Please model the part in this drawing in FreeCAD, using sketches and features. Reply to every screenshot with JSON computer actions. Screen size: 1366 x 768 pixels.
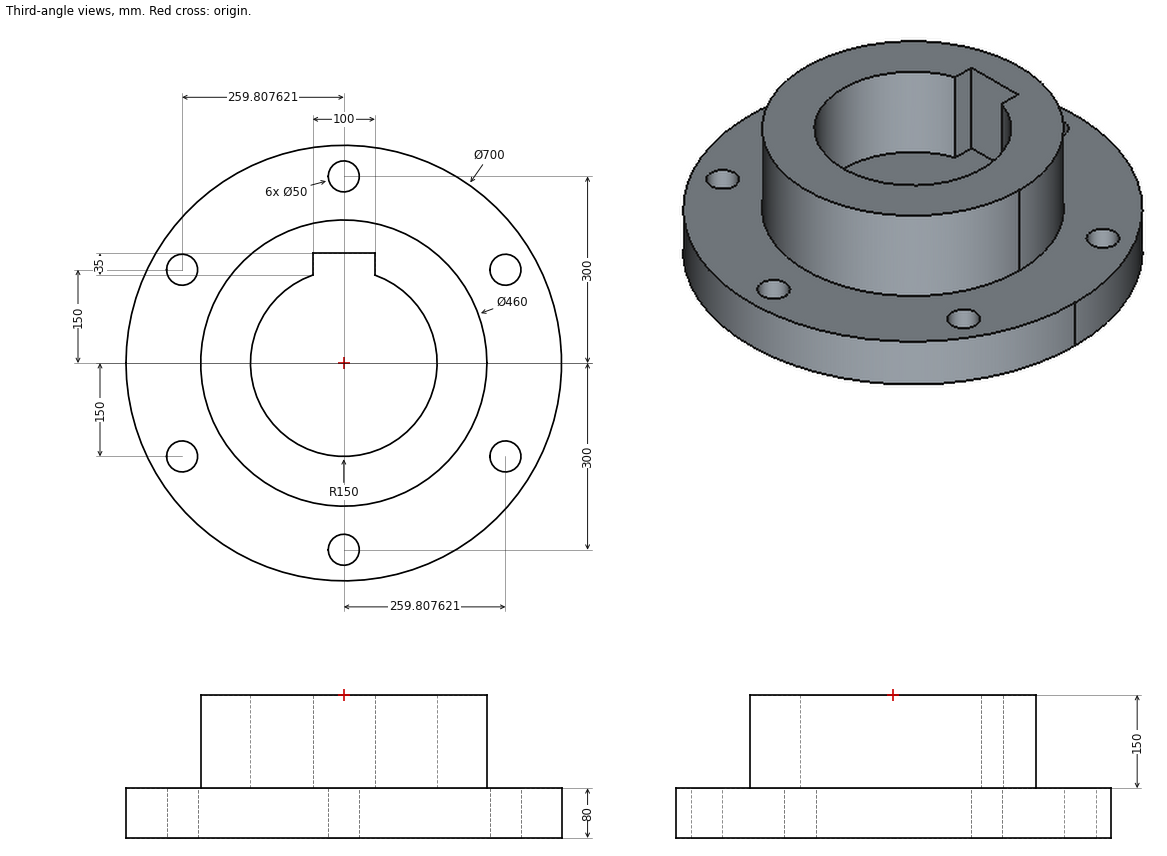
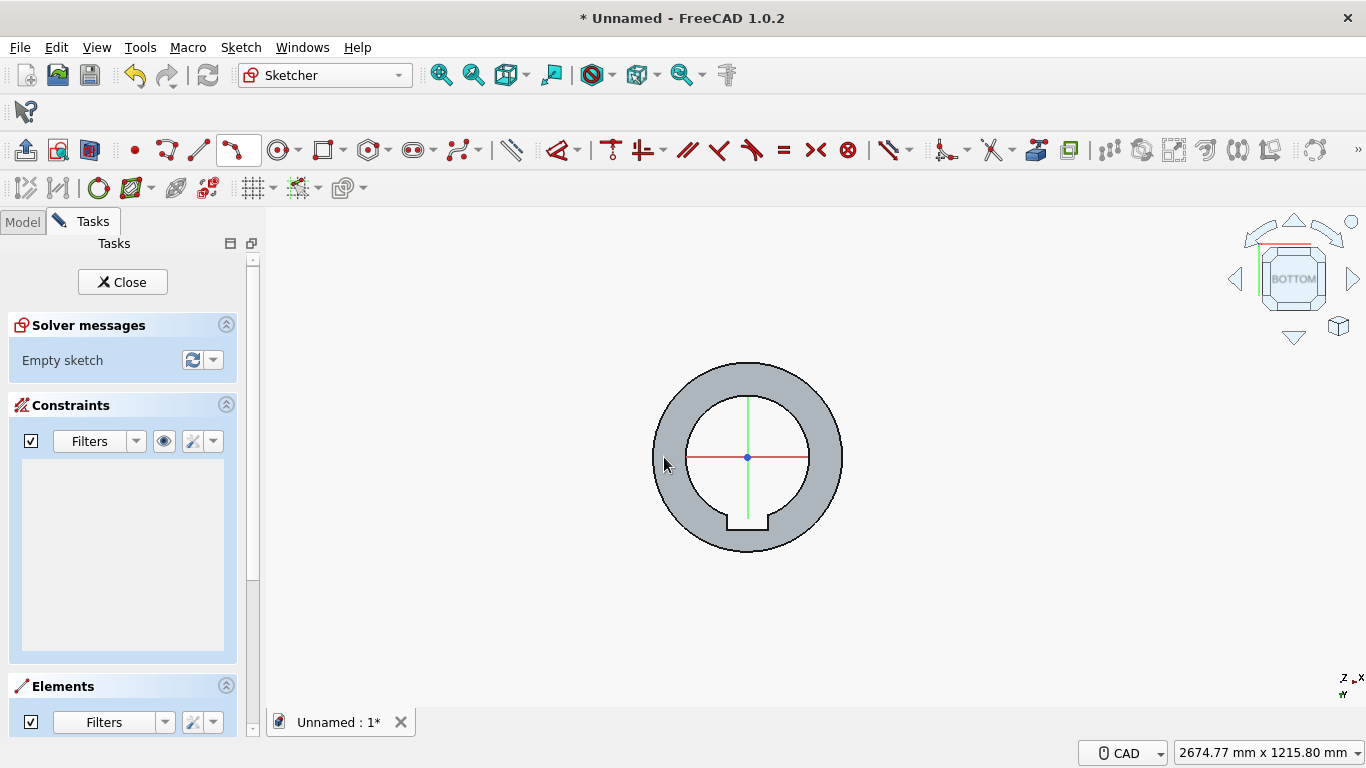
{"action": "left_click", "coordinate": [278, 150]}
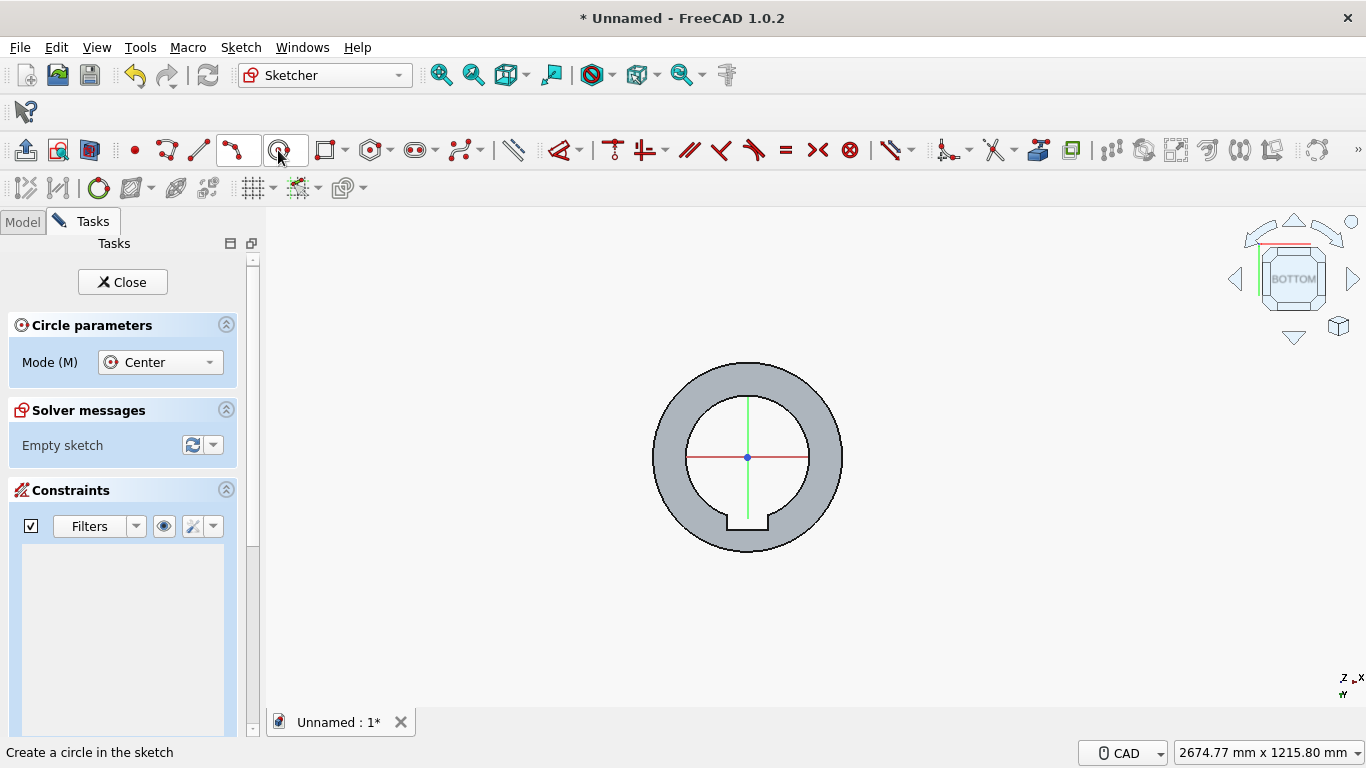
{"action": "left_click", "coordinate": [748, 457]}
{"action": "mouse_move", "coordinate": [849, 355]}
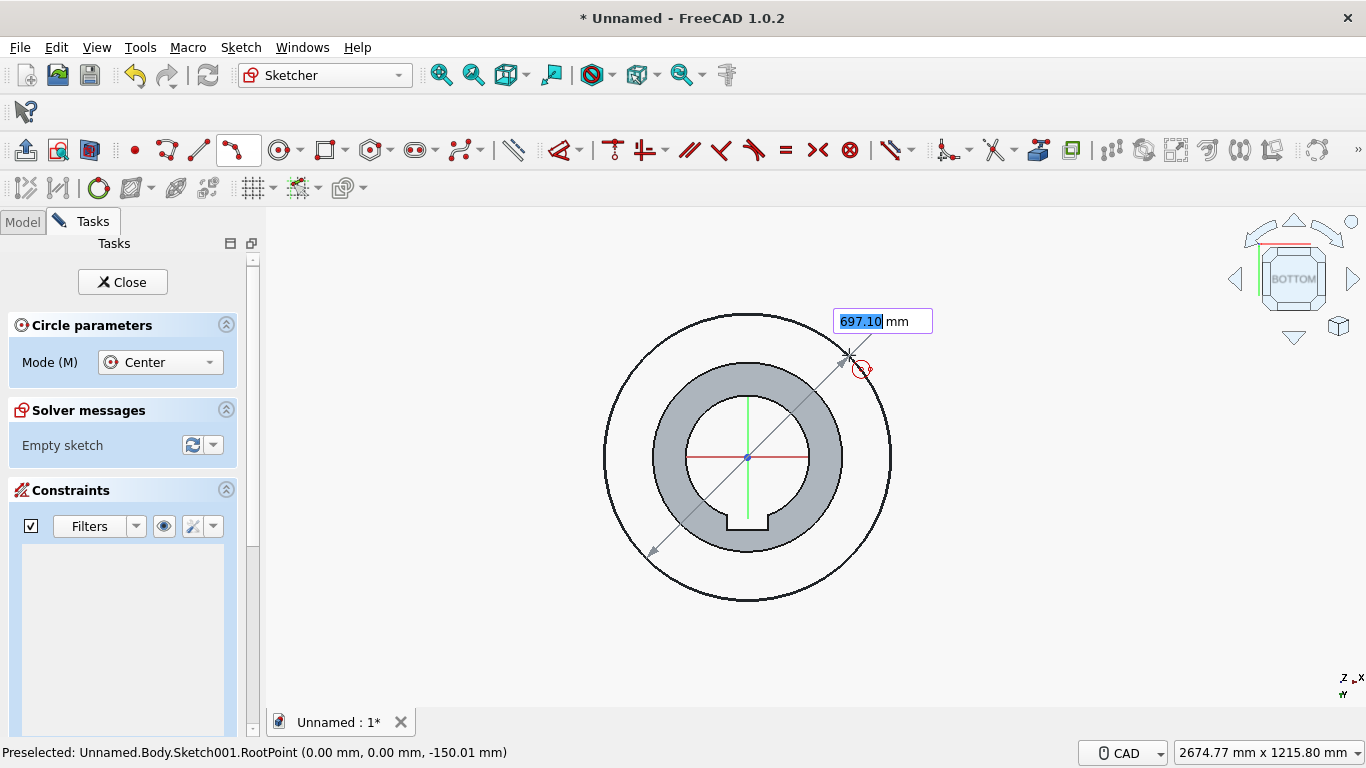
{"action": "type", "text": "700"}
{"action": "key", "text": "Return"}
{"action": "key", "text": "Escape"}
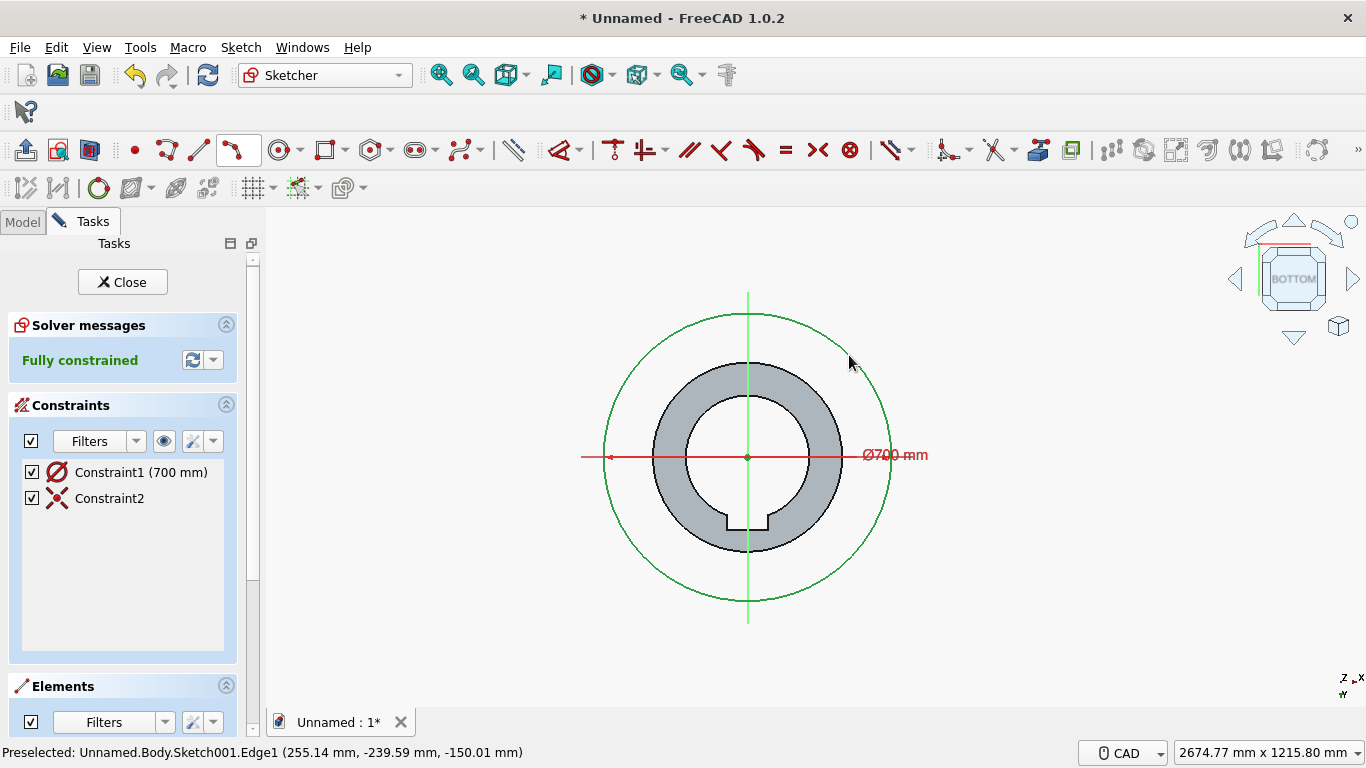
{"action": "left_click", "coordinate": [123, 282]}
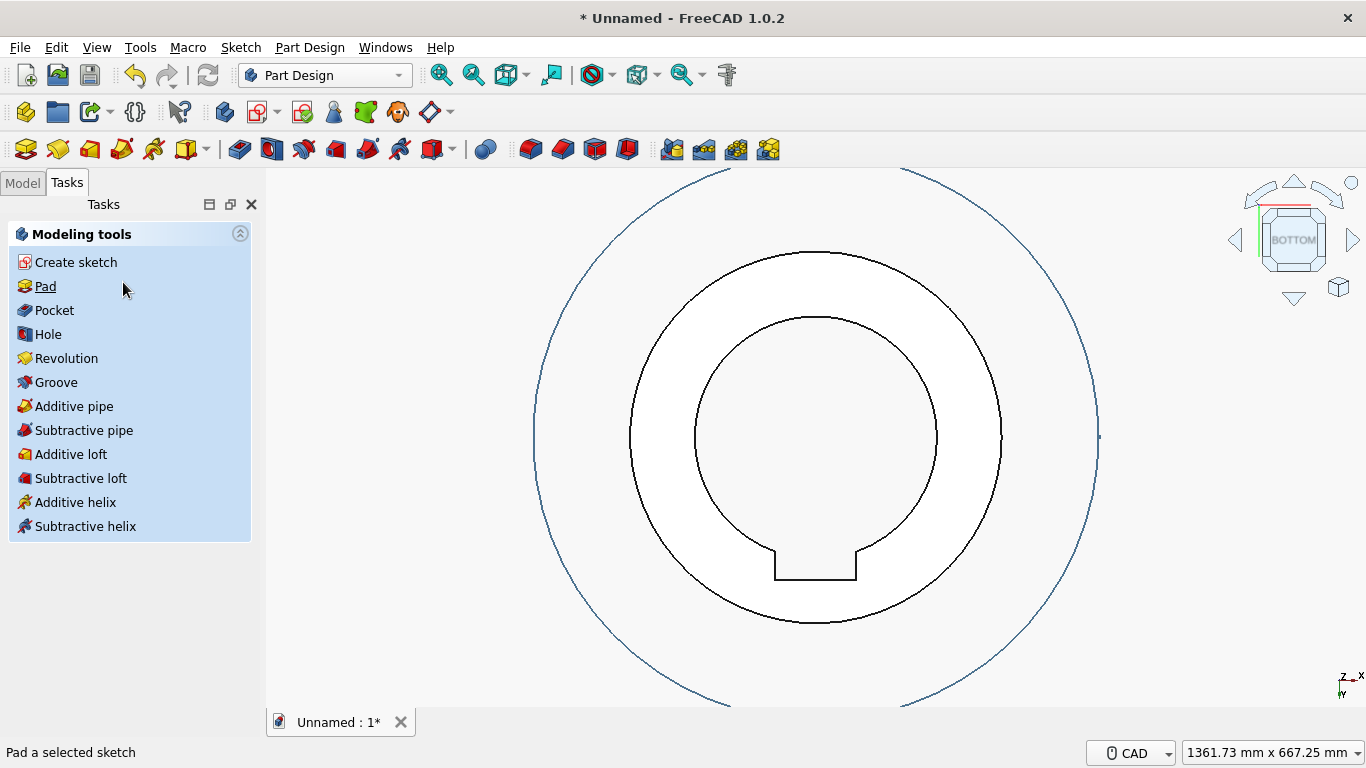
{"action": "left_click", "coordinate": [26, 150]}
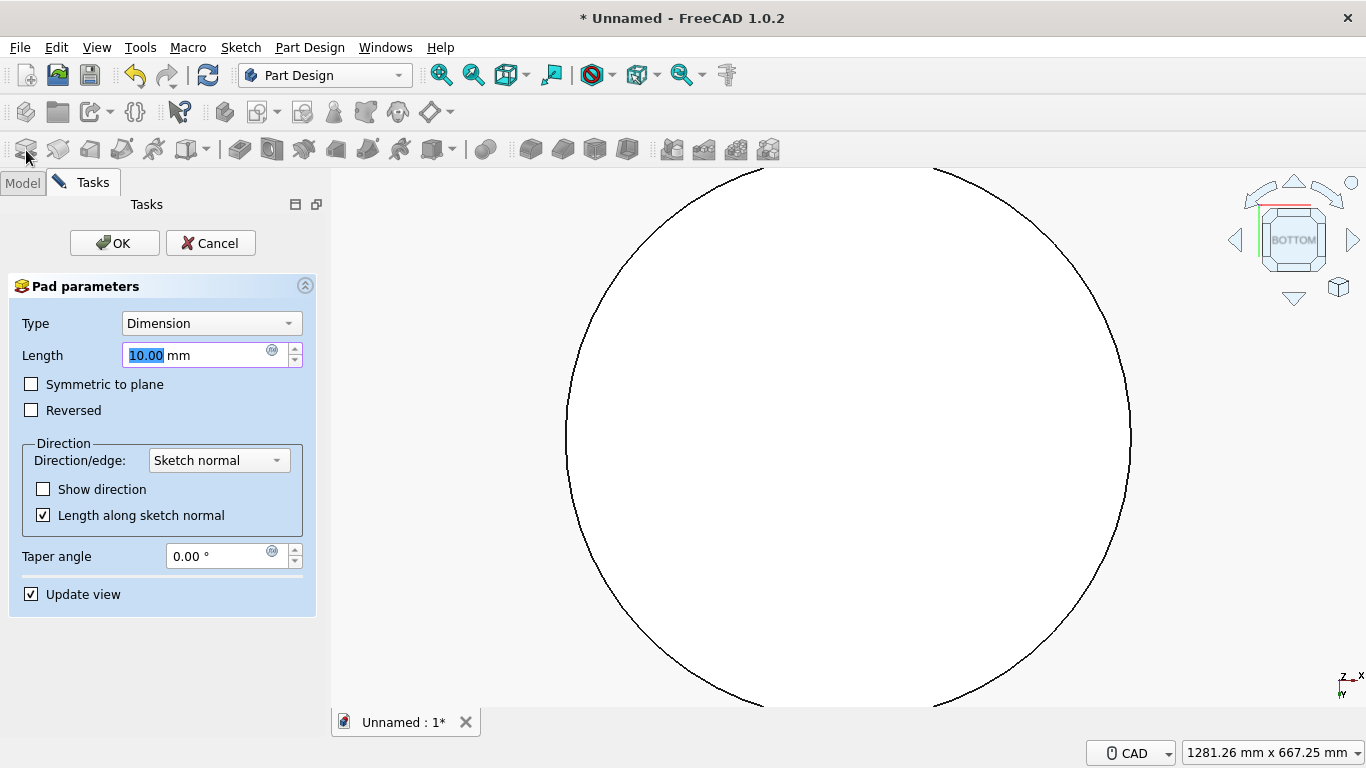
{"action": "type", "text": "80"}
{"action": "key", "text": "Tab"}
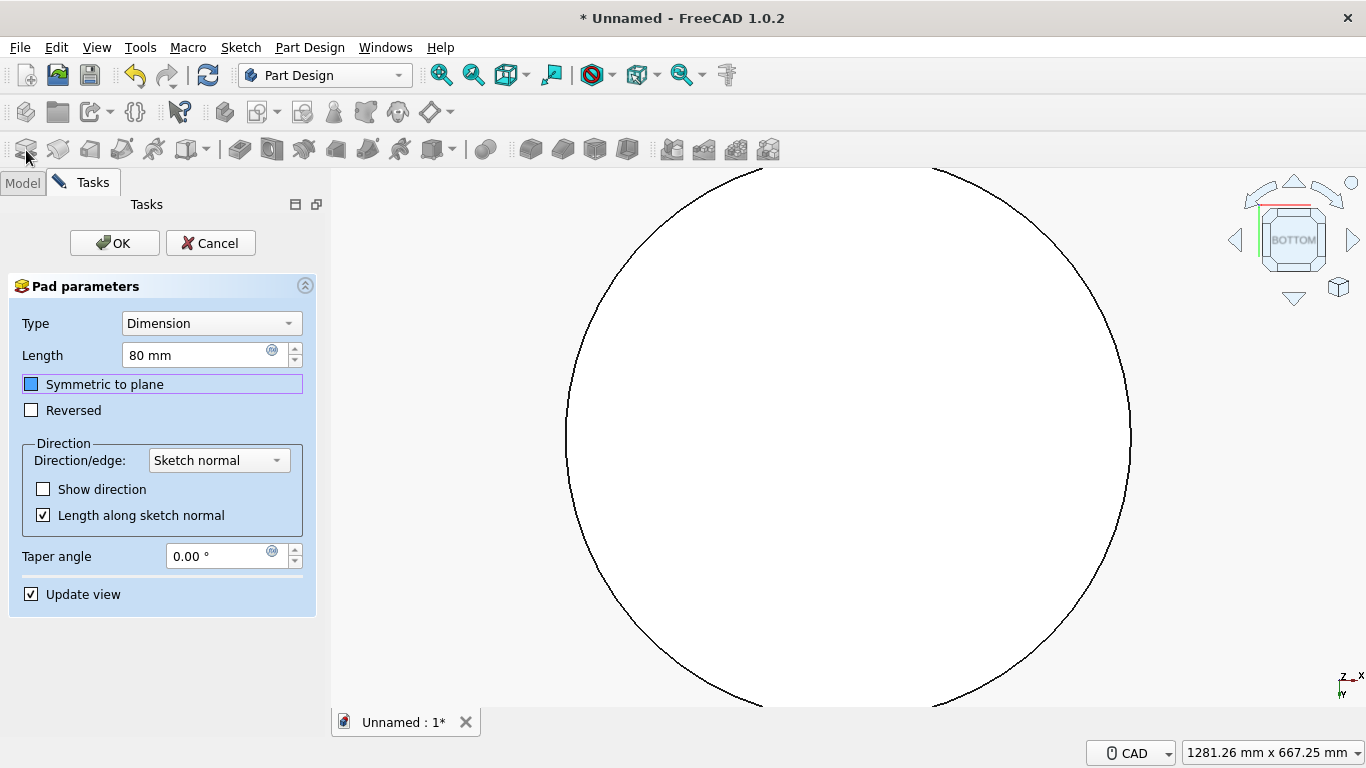
{"action": "left_click", "coordinate": [115, 243]}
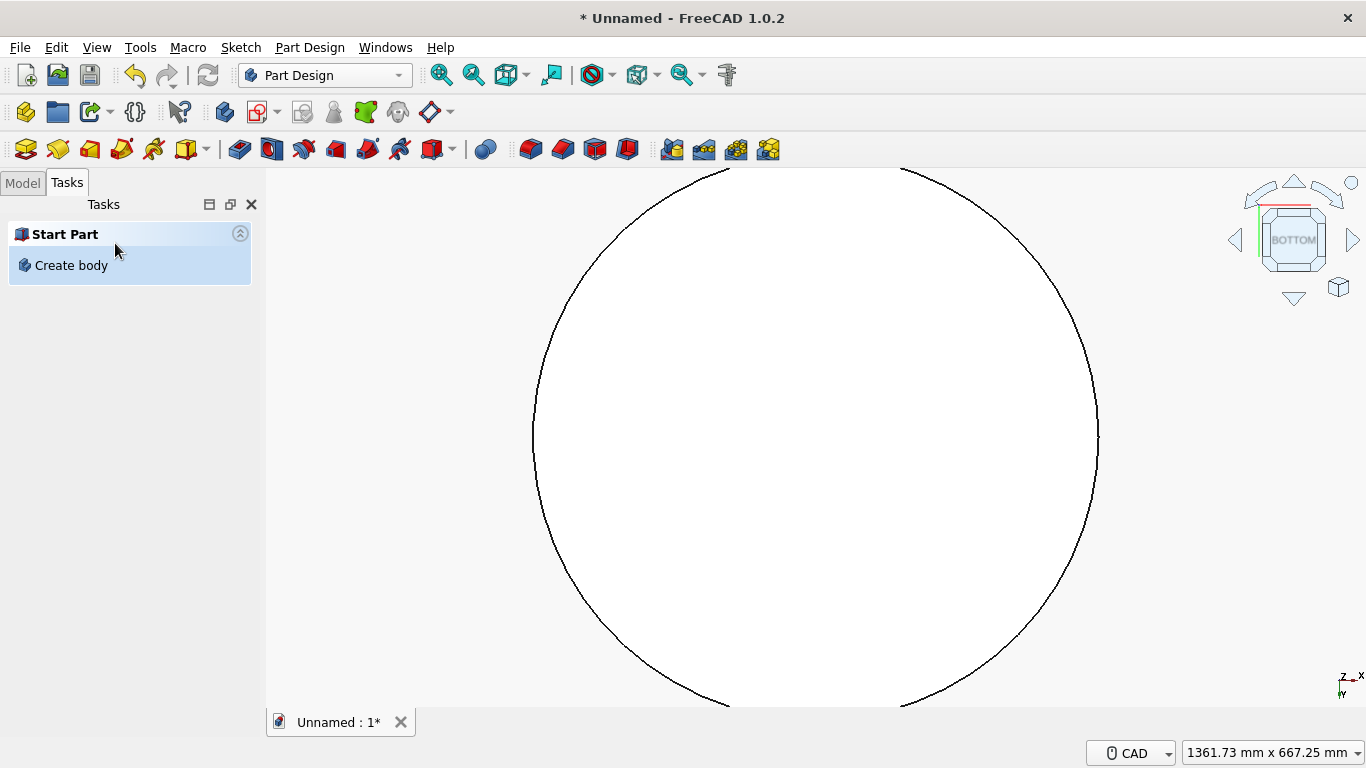
{"action": "key", "text": "v f"}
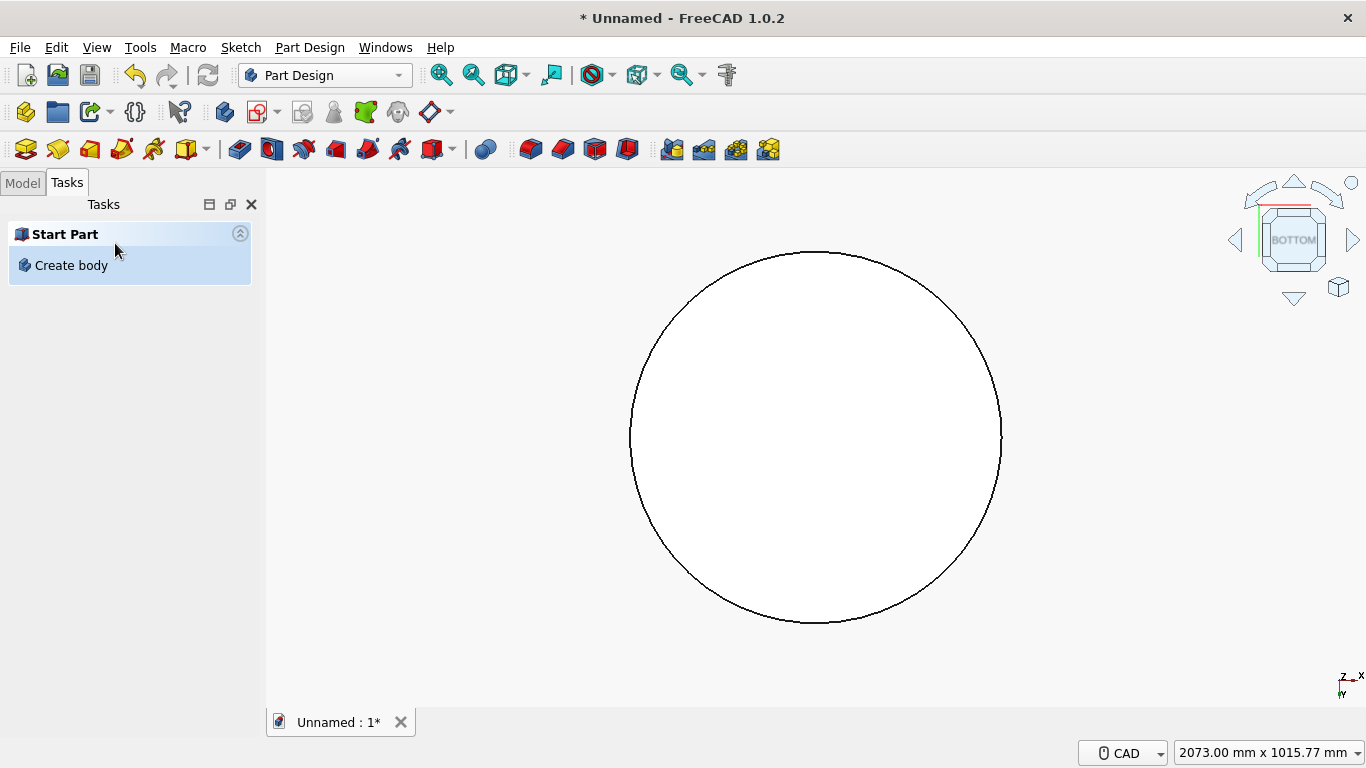
{"action": "left_click", "coordinate": [816, 436]}